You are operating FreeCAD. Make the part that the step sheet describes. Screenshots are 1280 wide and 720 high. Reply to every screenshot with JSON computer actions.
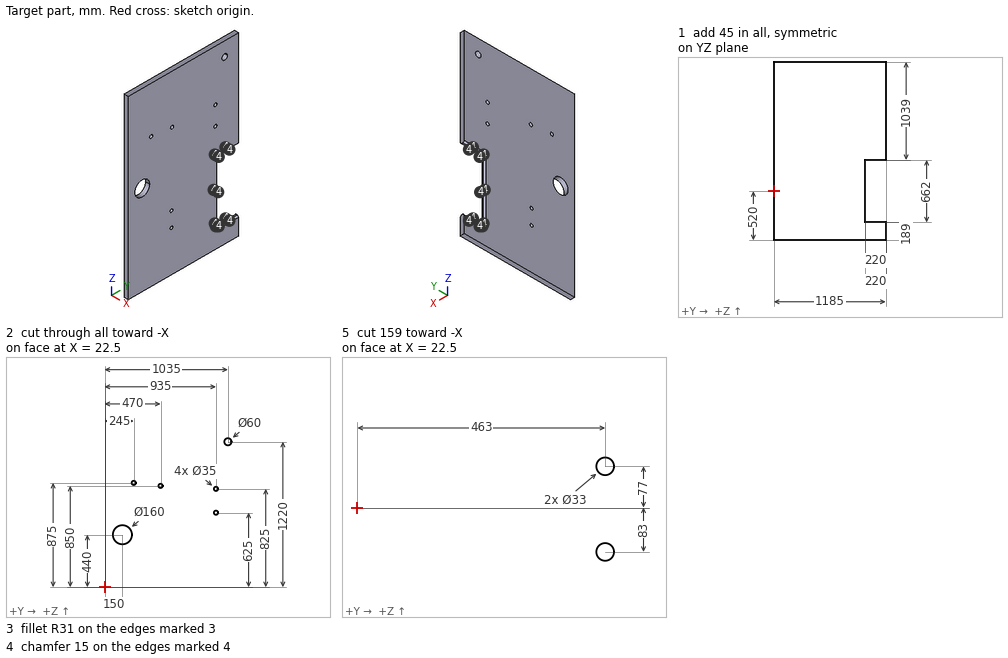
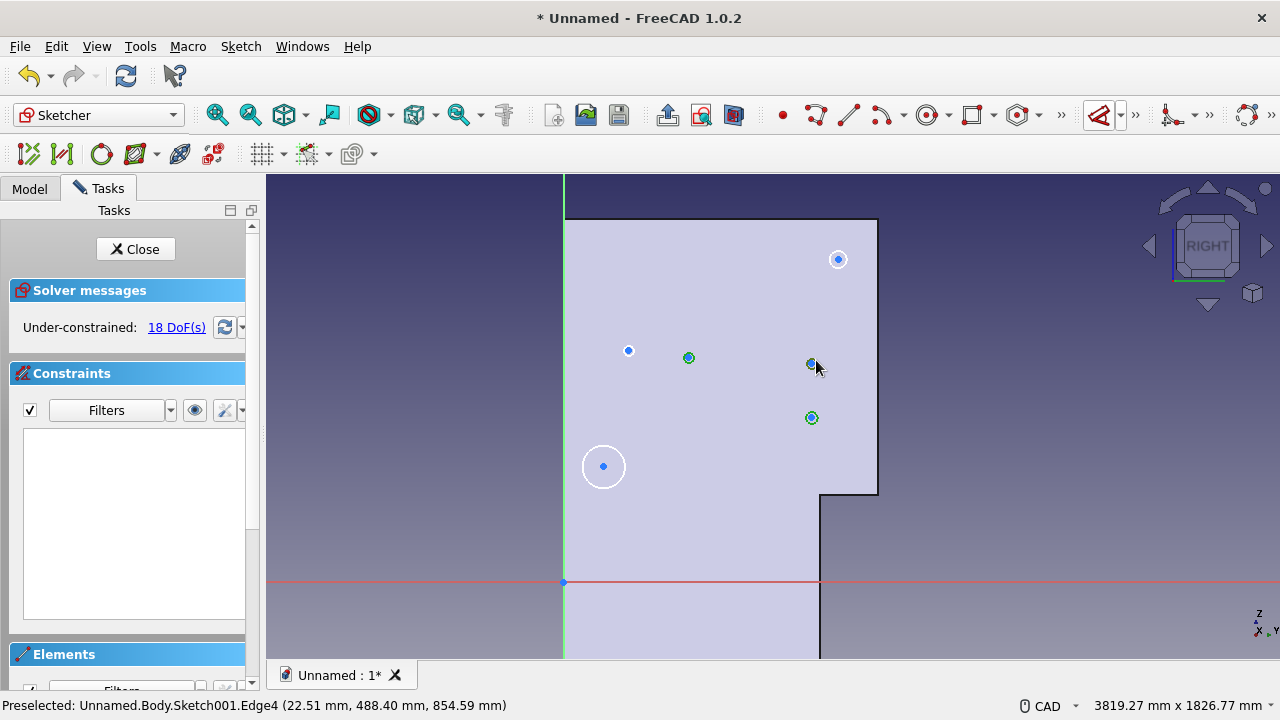
{"action": "scroll", "coordinate": [632, 347], "scroll_direction": "up", "scroll_amount": 6}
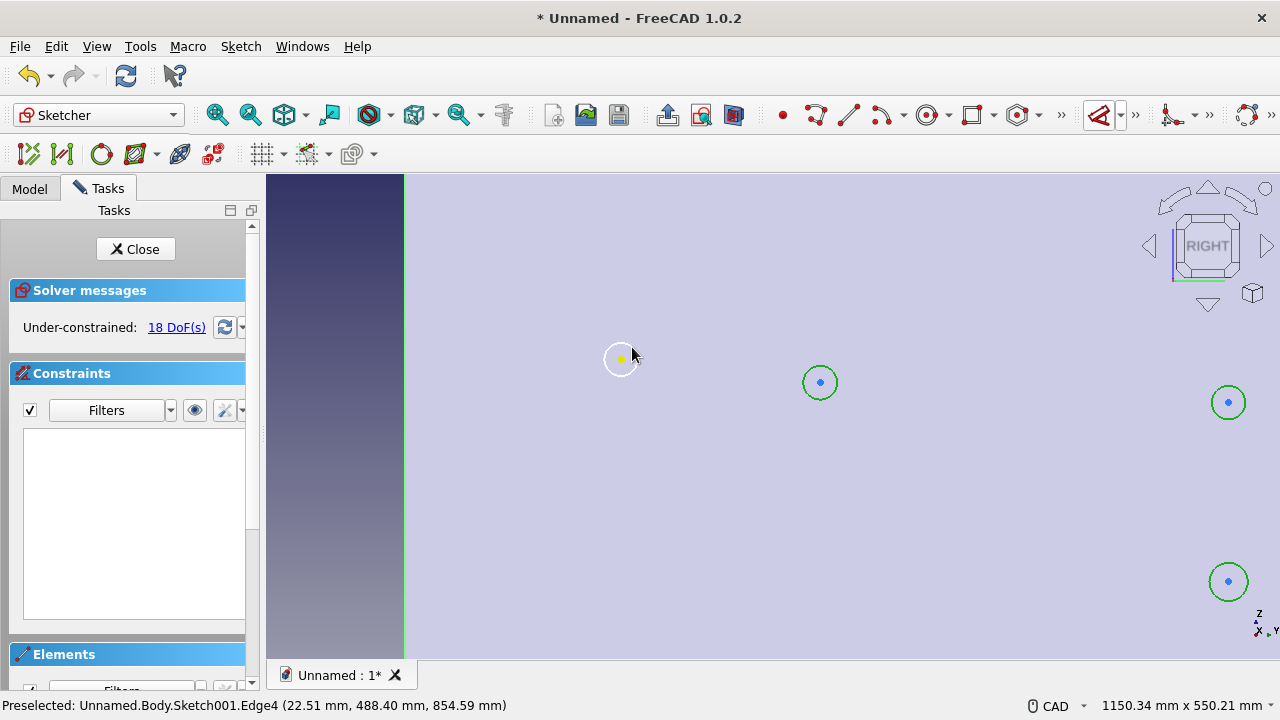
{"action": "left_click", "coordinate": [633, 348]}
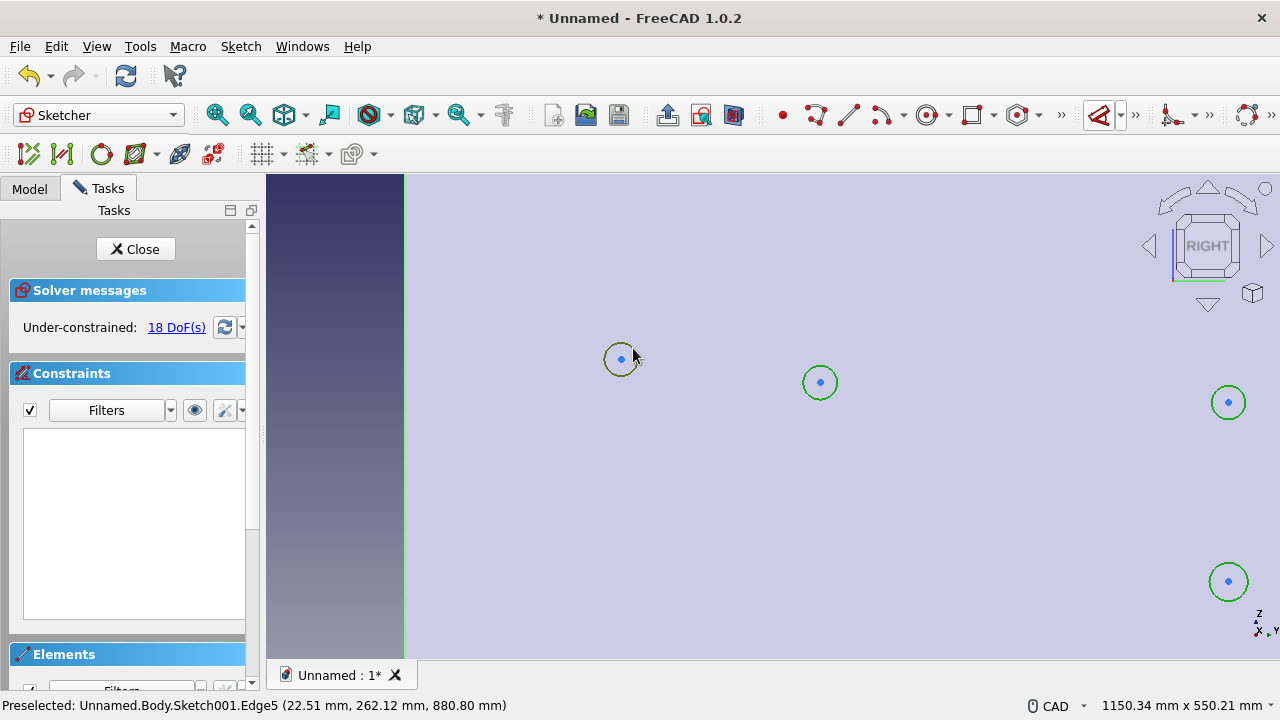
{"action": "key", "text": "e"}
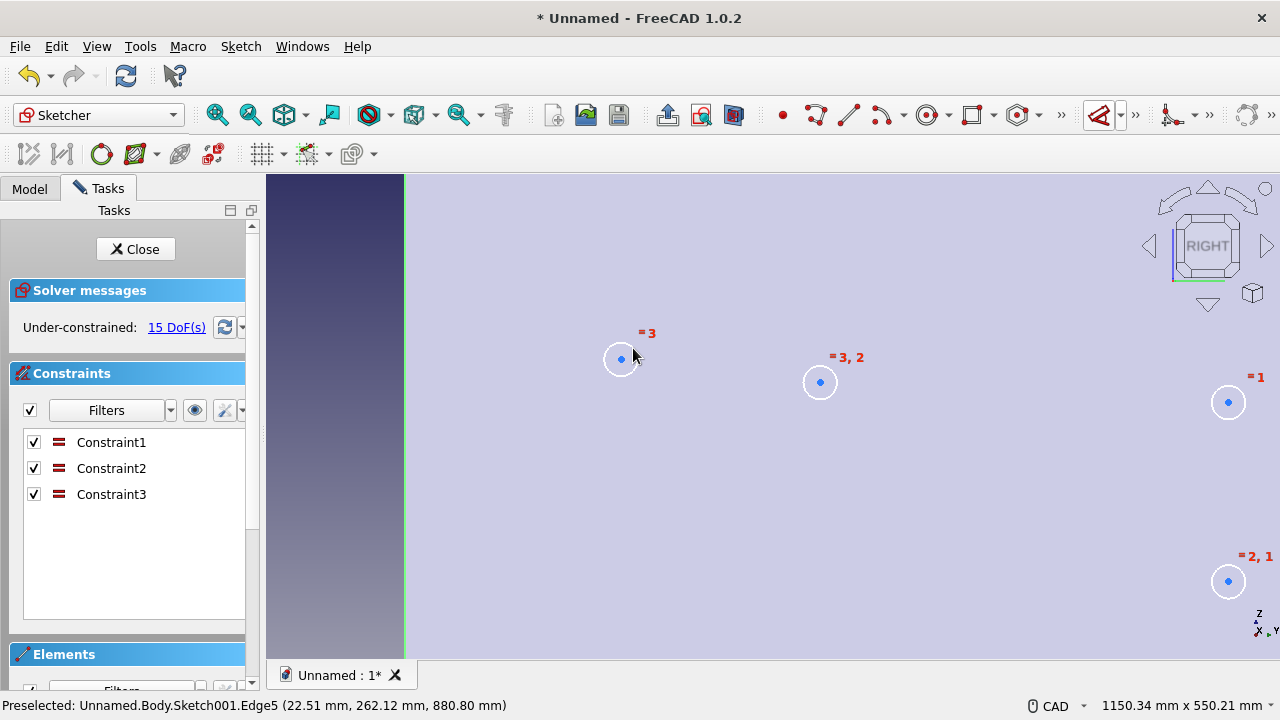
{"action": "scroll", "coordinate": [631, 347], "scroll_direction": "down", "scroll_amount": 6}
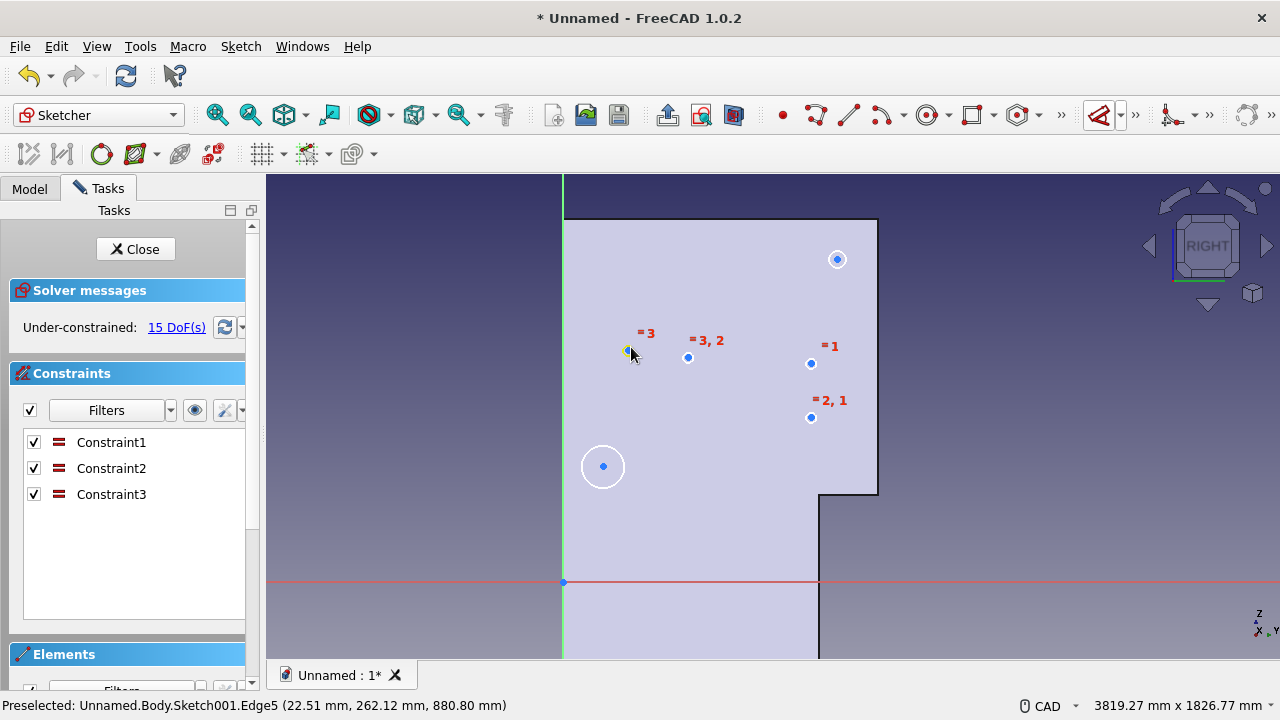
{"action": "left_click", "coordinate": [811, 364]}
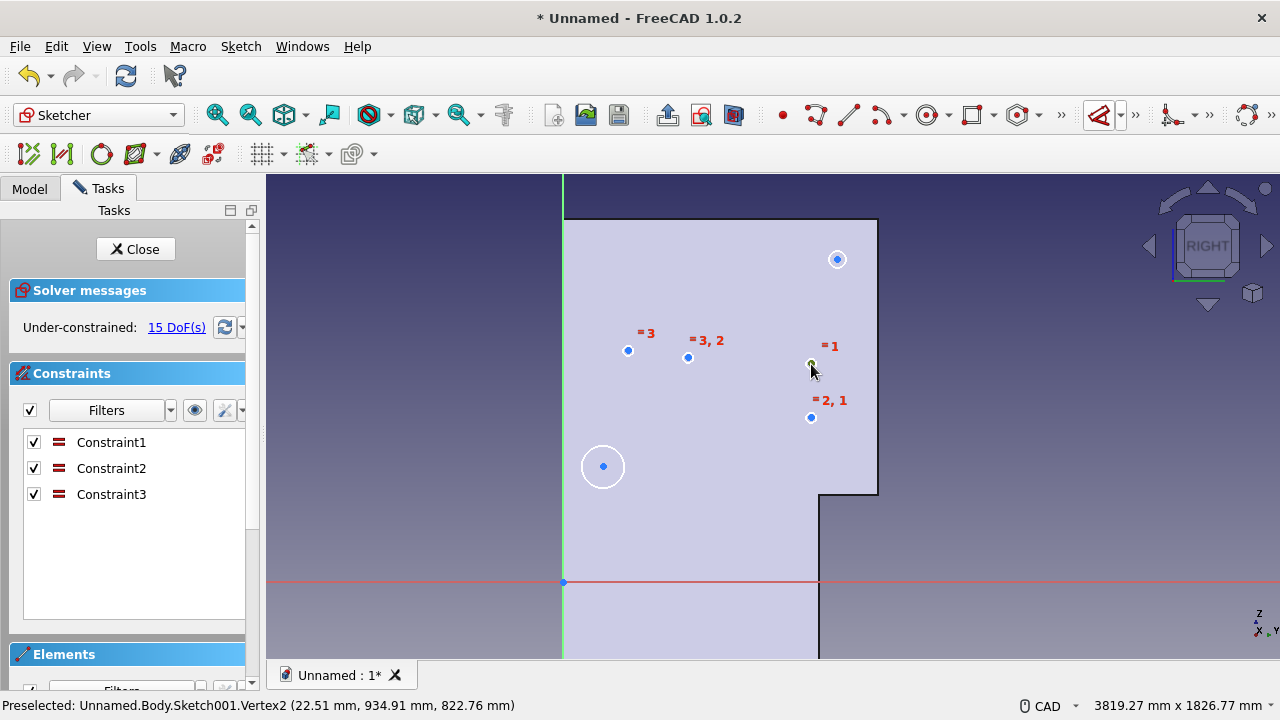
{"action": "left_click", "coordinate": [811, 418]}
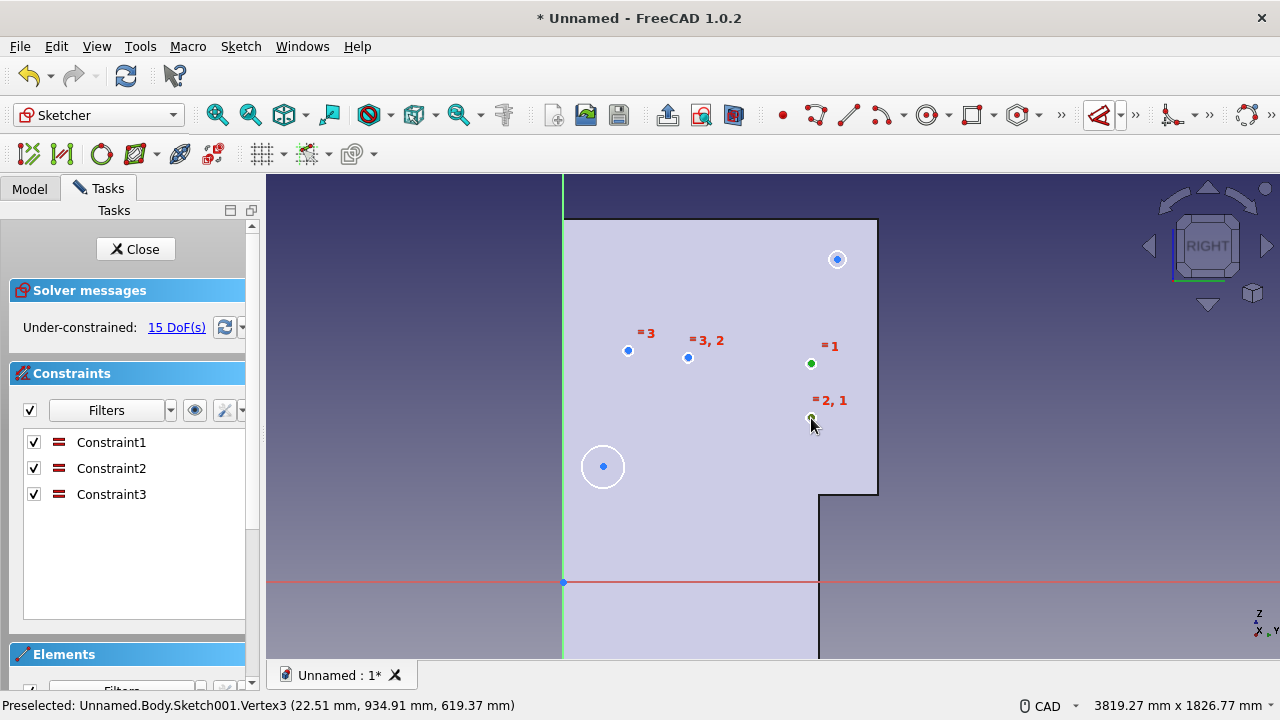
{"action": "key", "text": "v"}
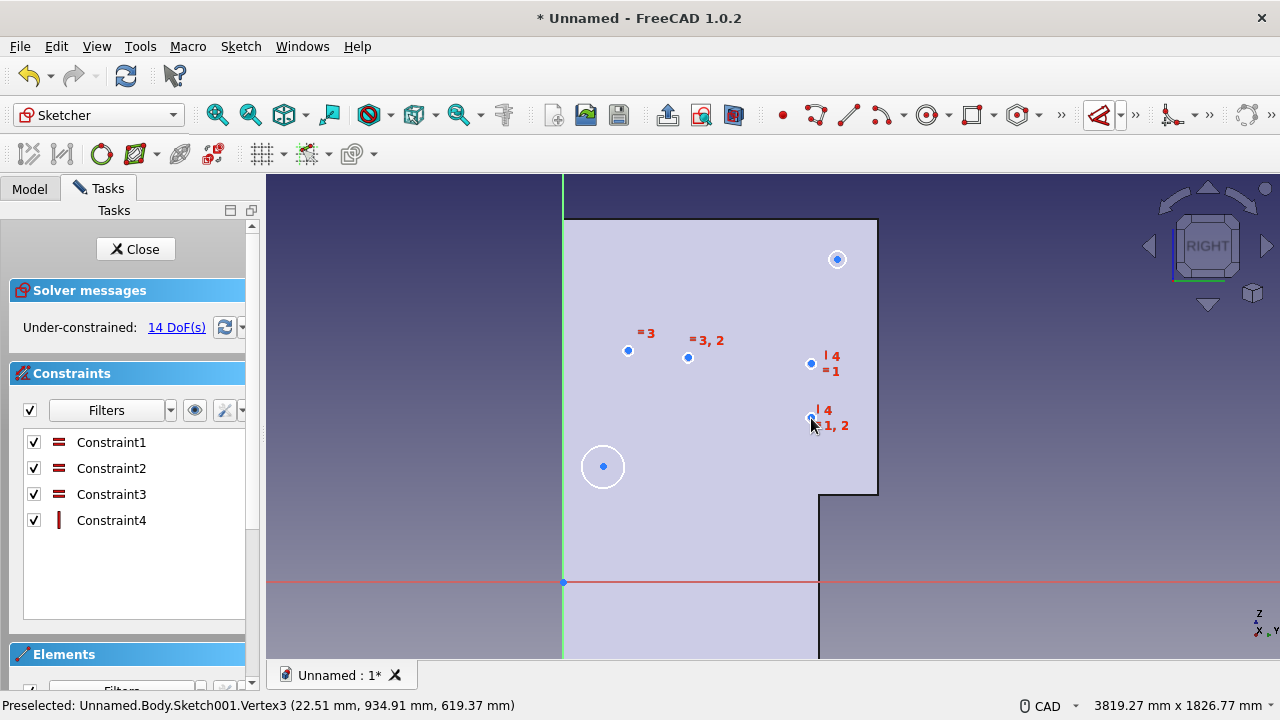
{"action": "scroll", "coordinate": [829, 259], "scroll_direction": "up", "scroll_amount": 5}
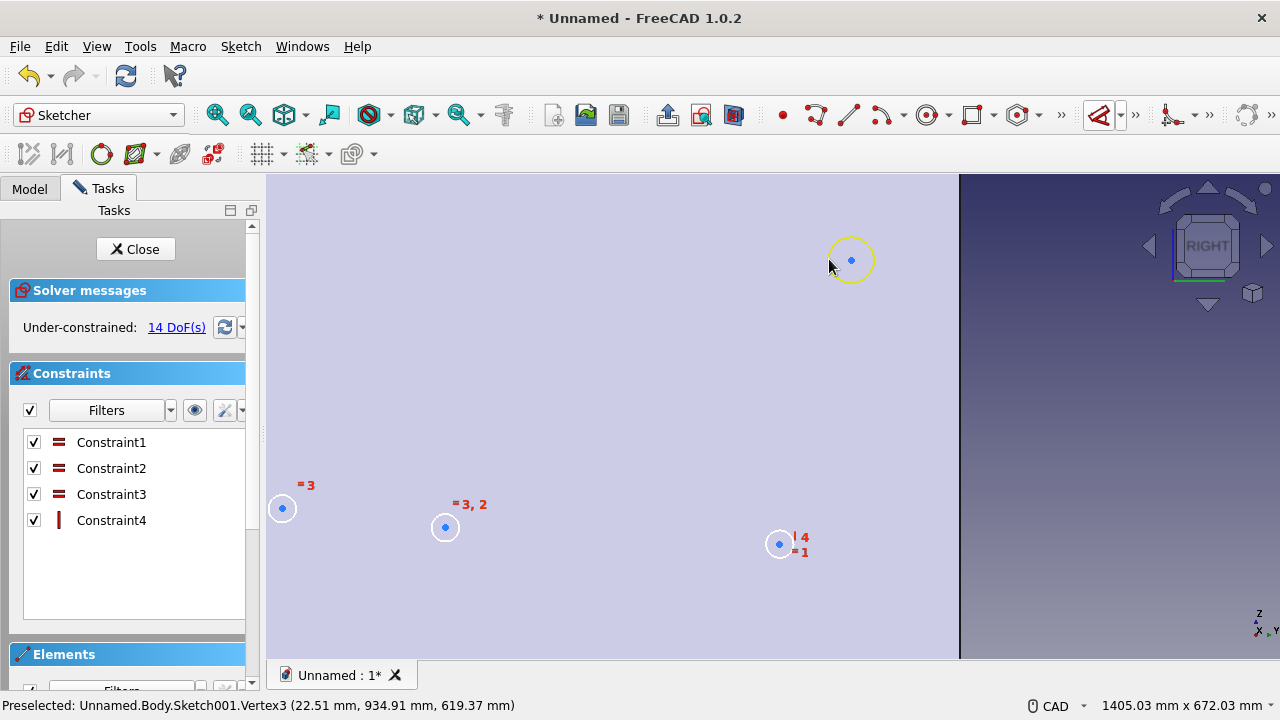
{"action": "left_click", "coordinate": [828, 260]}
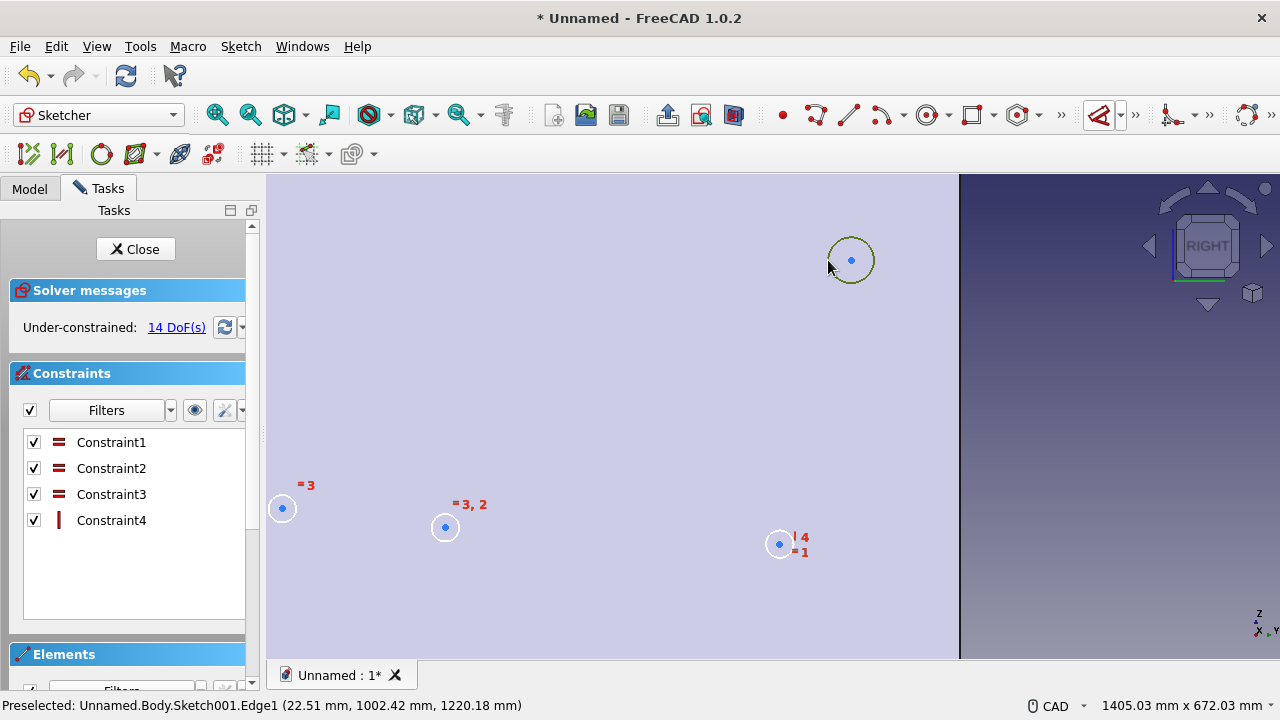
{"action": "key", "text": "k o"}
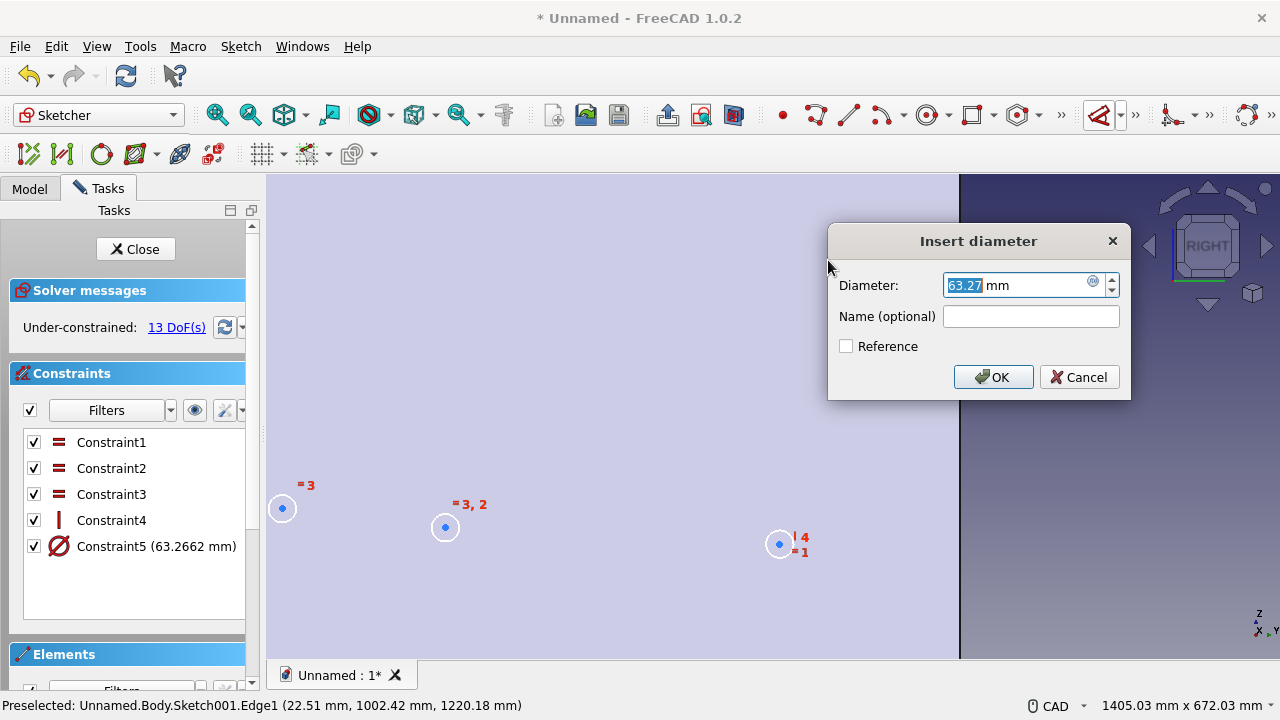
{"action": "type", "text": "60"}
{"action": "key", "text": "Return"}